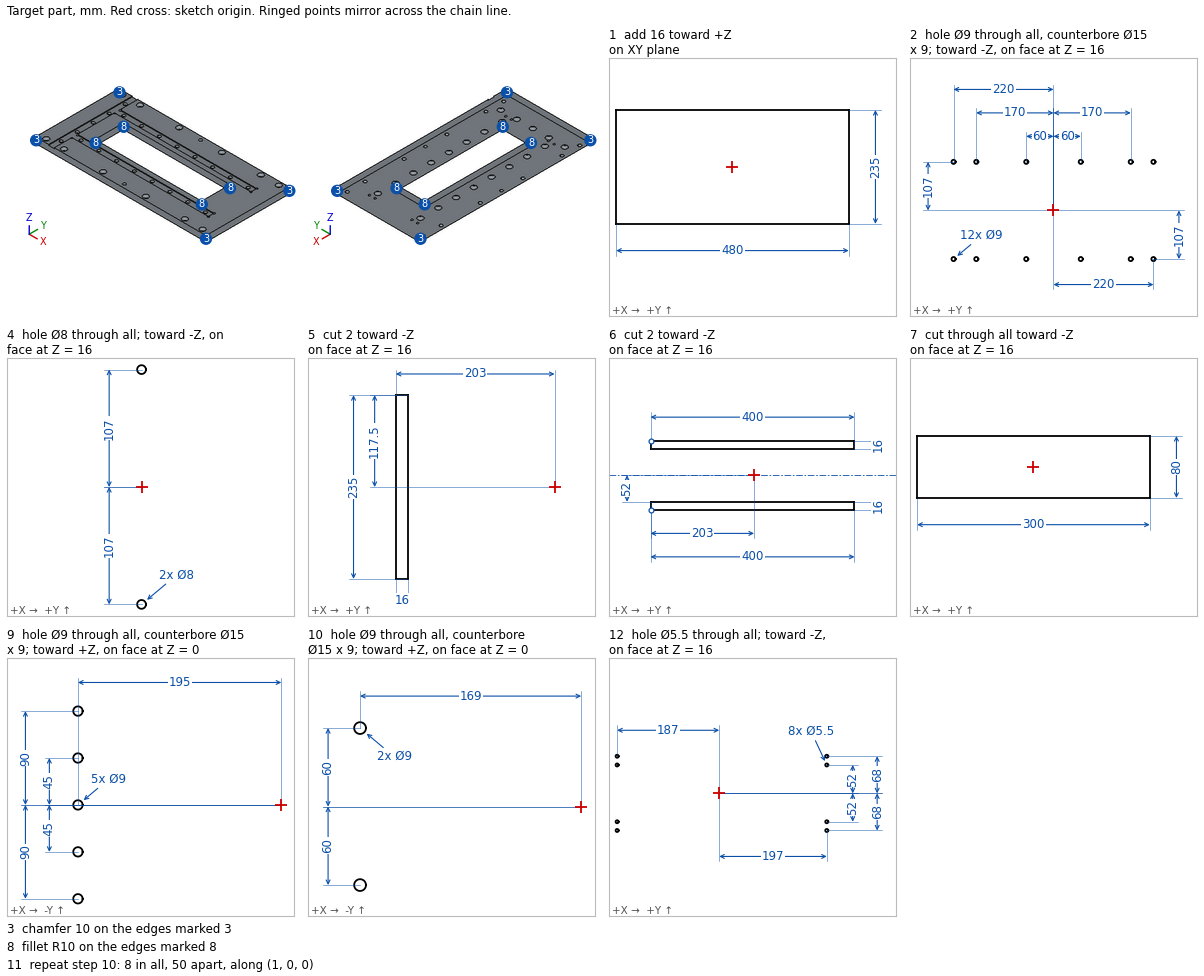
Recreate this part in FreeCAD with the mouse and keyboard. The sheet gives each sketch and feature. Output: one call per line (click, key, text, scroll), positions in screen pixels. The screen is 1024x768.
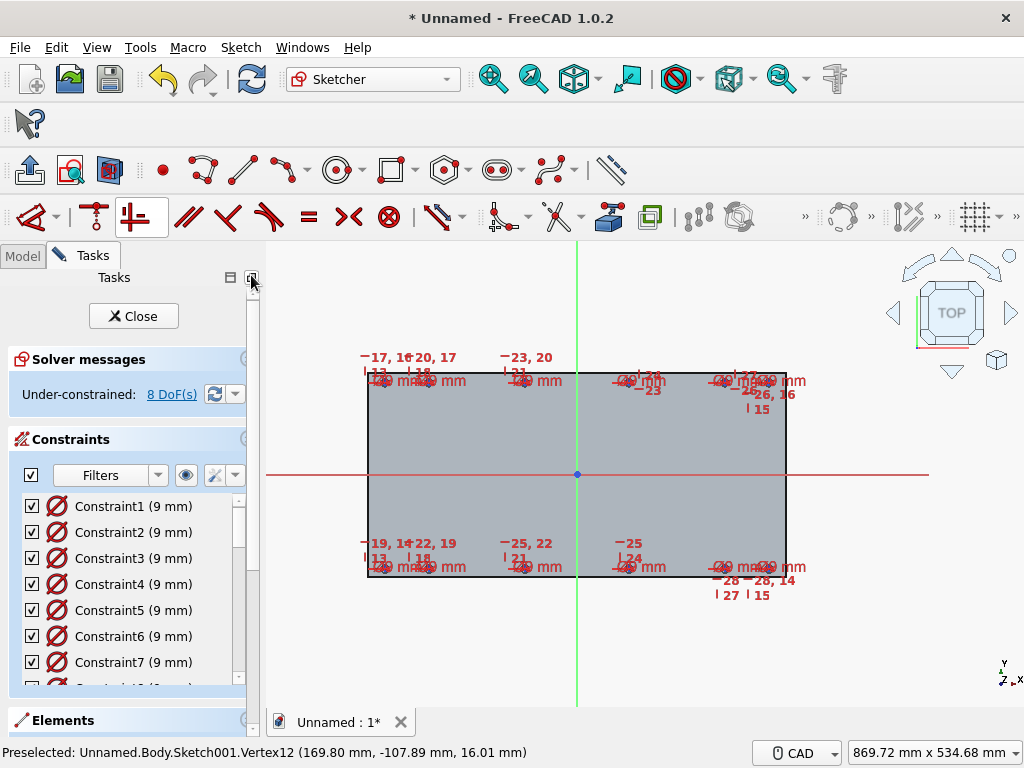
click(32, 218)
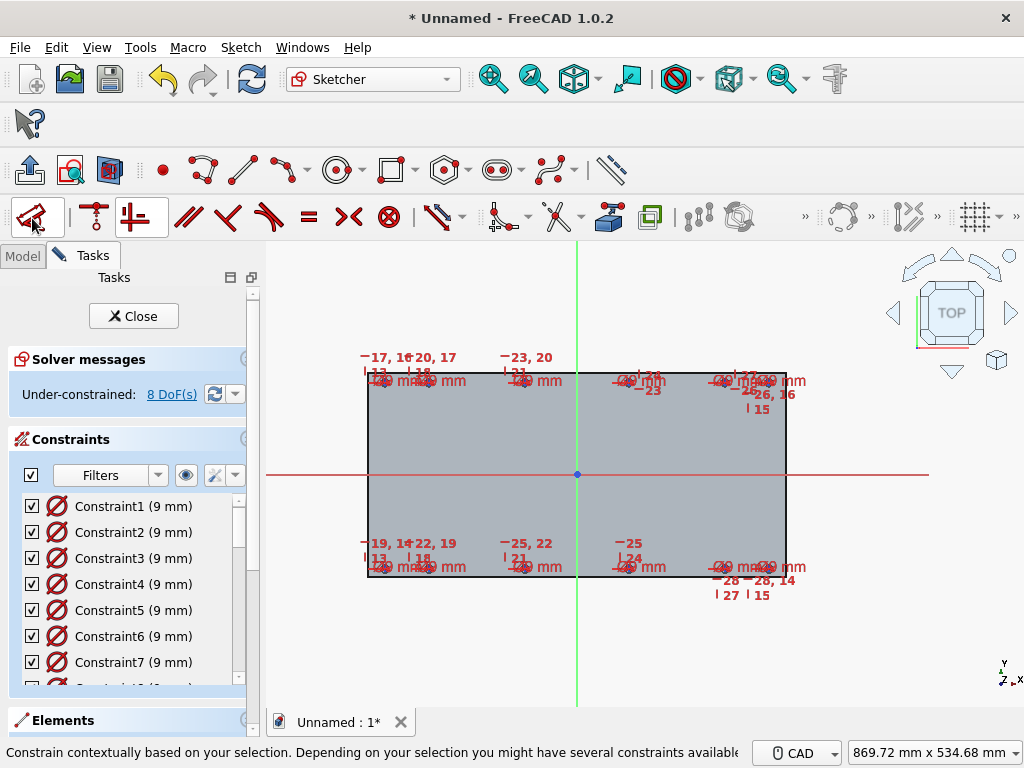
click(525, 383)
click(551, 349)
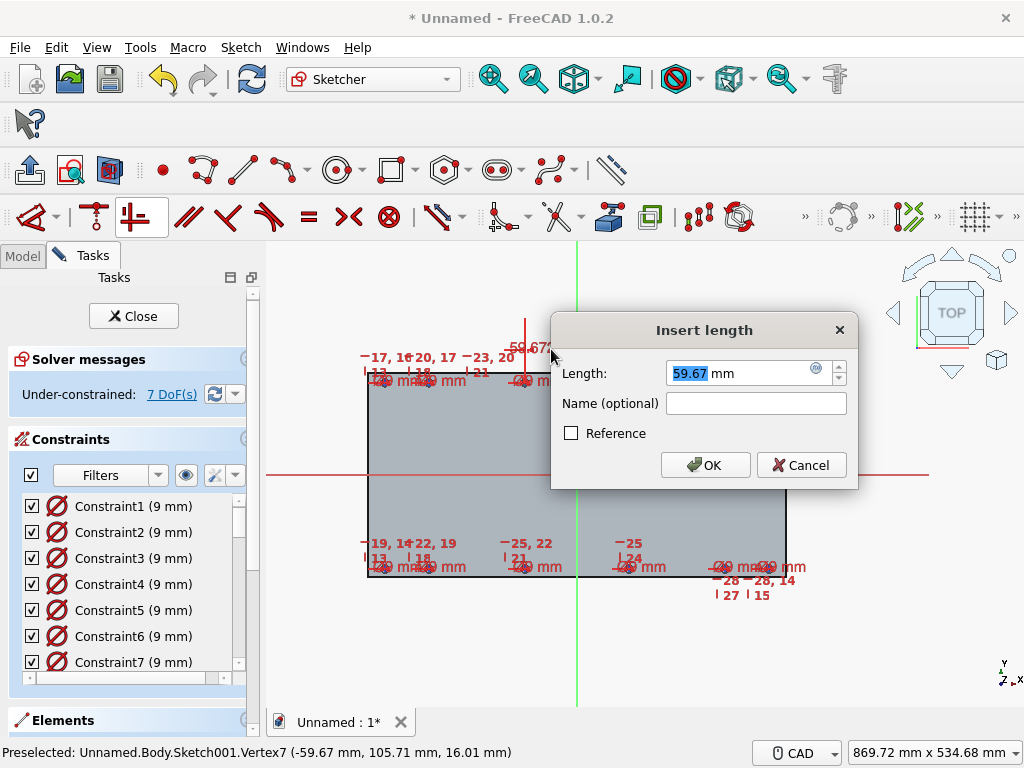
text(60)
key(Return)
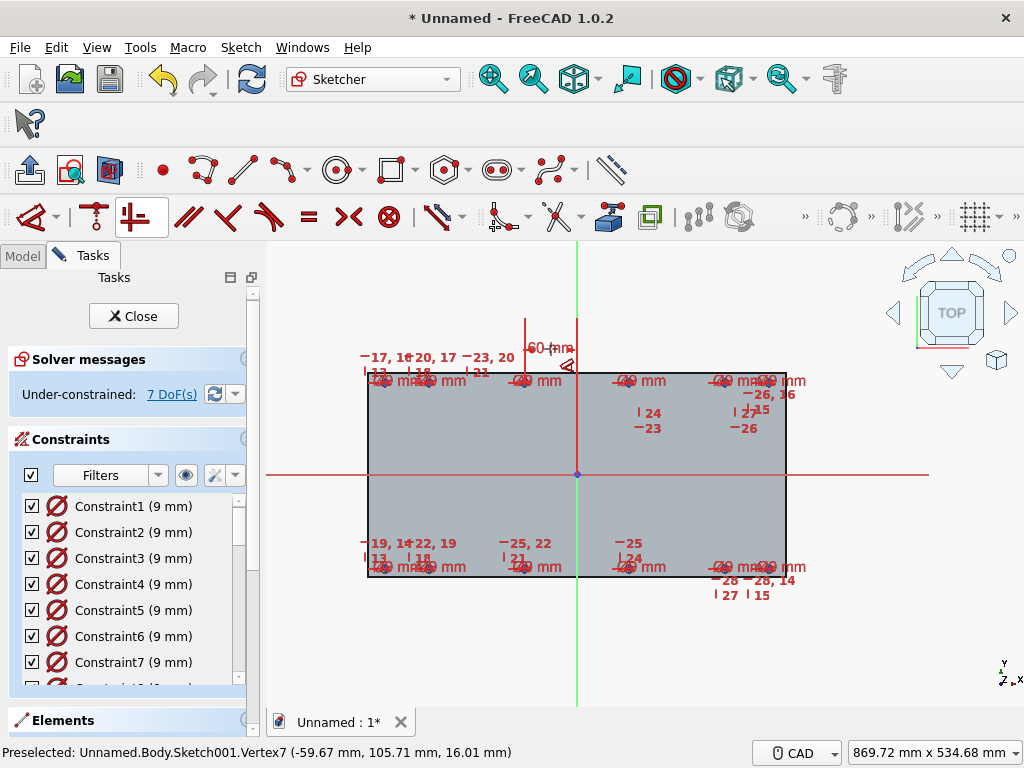
click(629, 383)
click(621, 349)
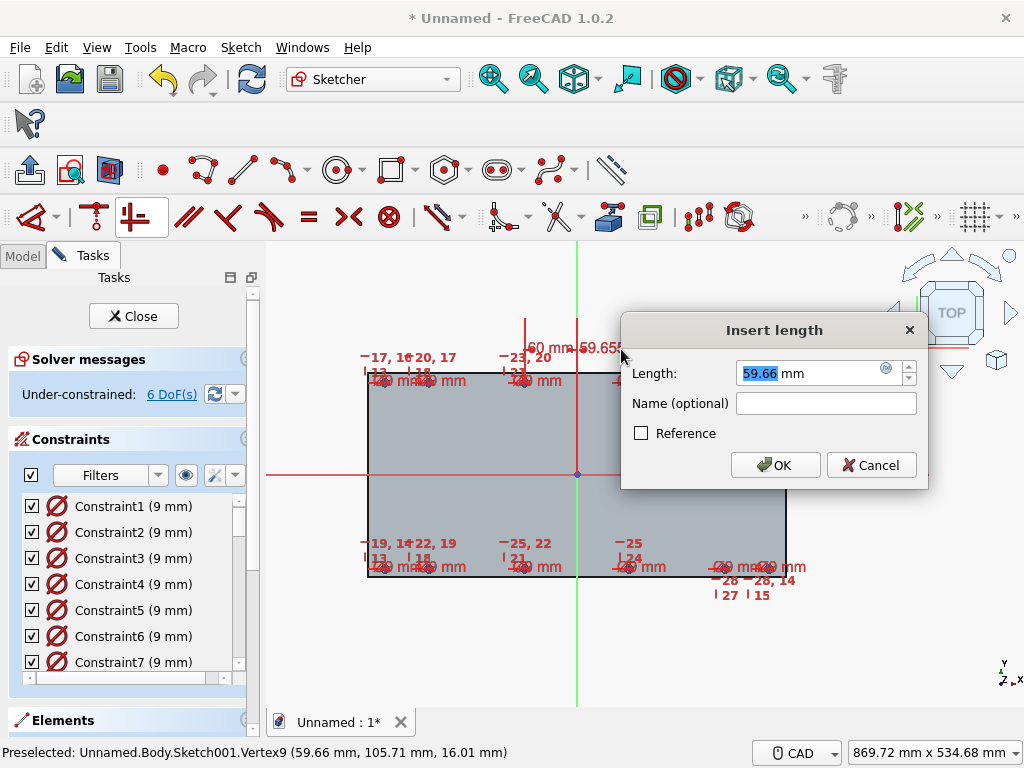
text(60)
key(Return)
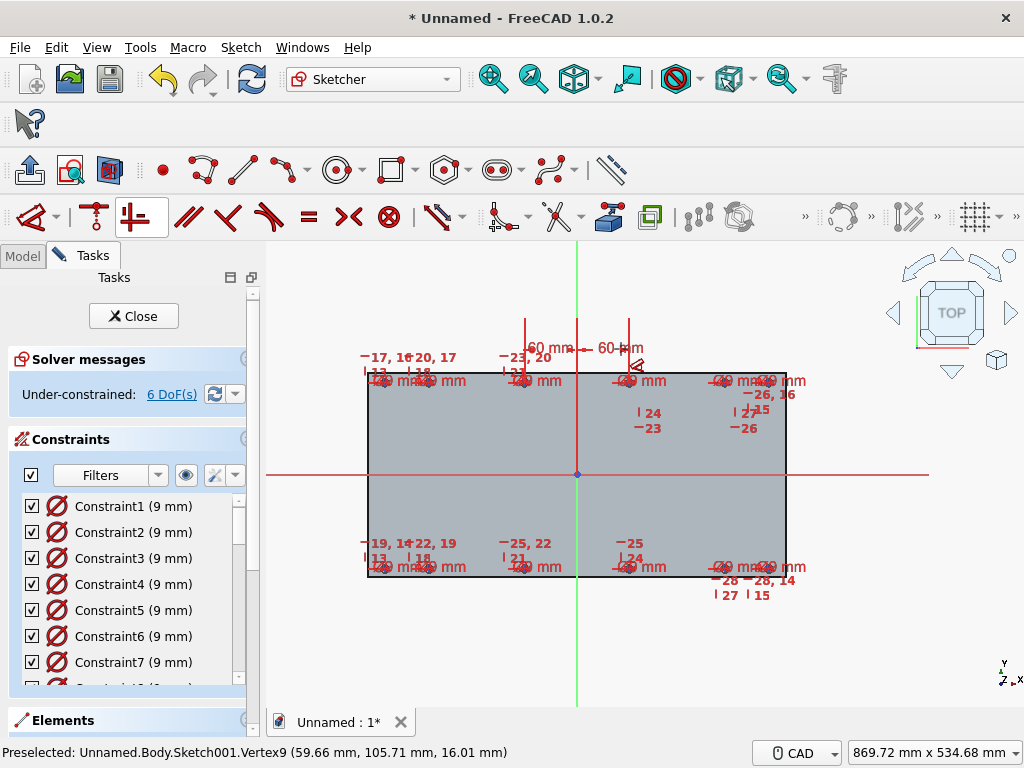
click(385, 383)
click(437, 349)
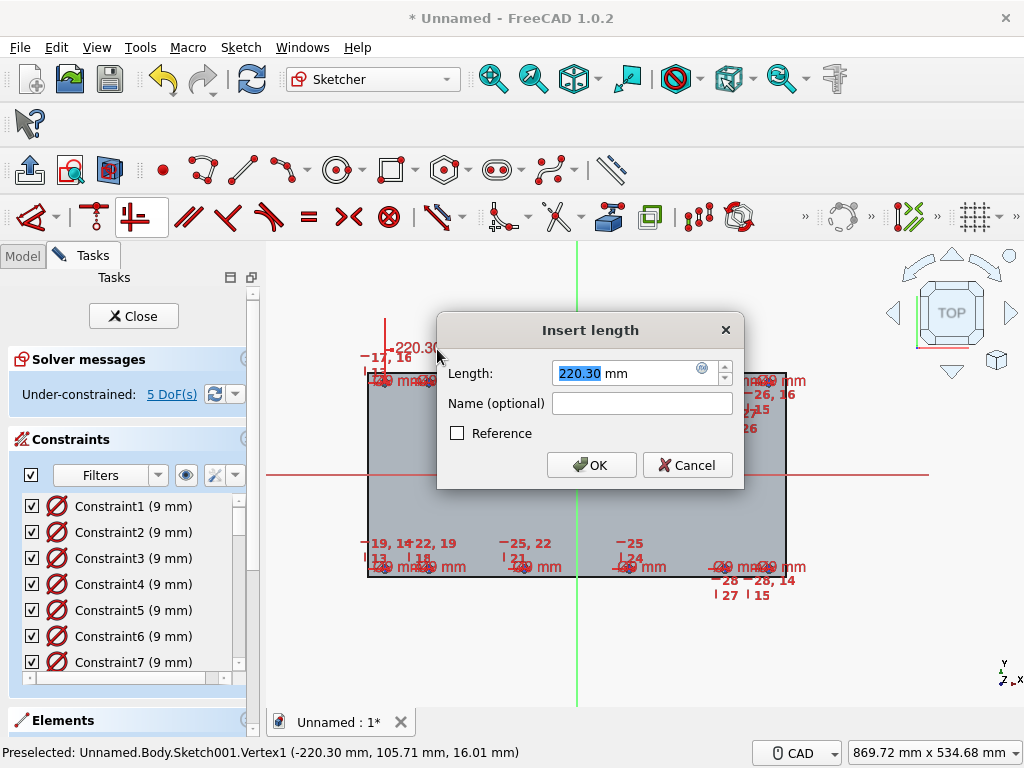
text(220)
key(Return)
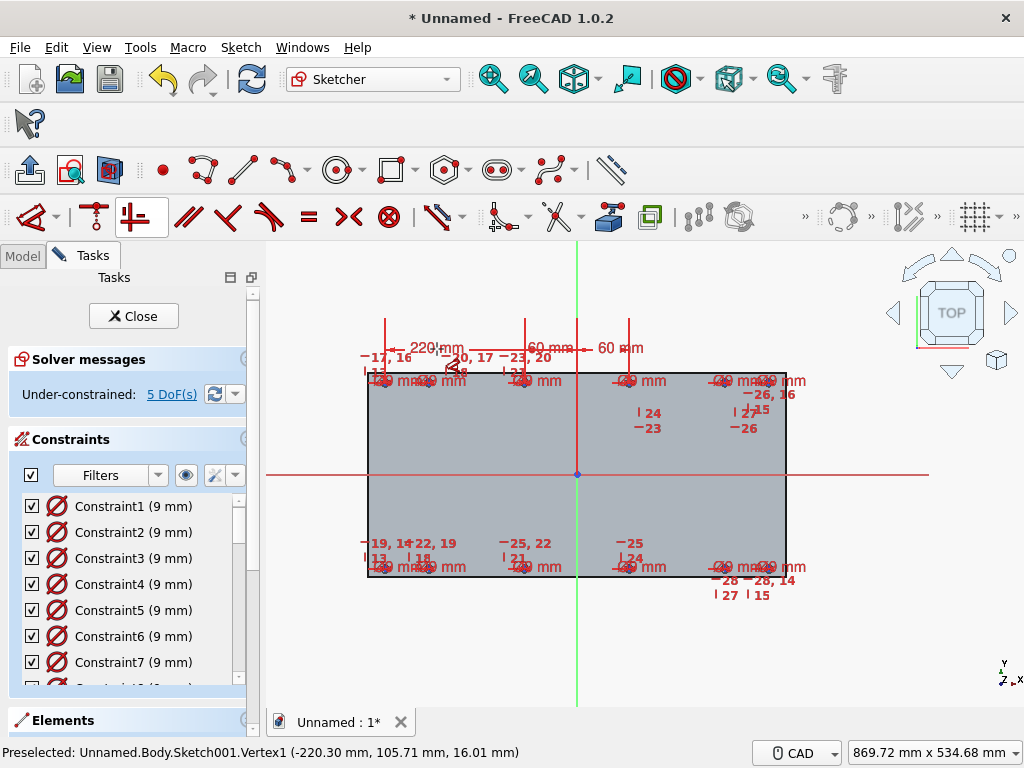
click(385, 383)
click(351, 429)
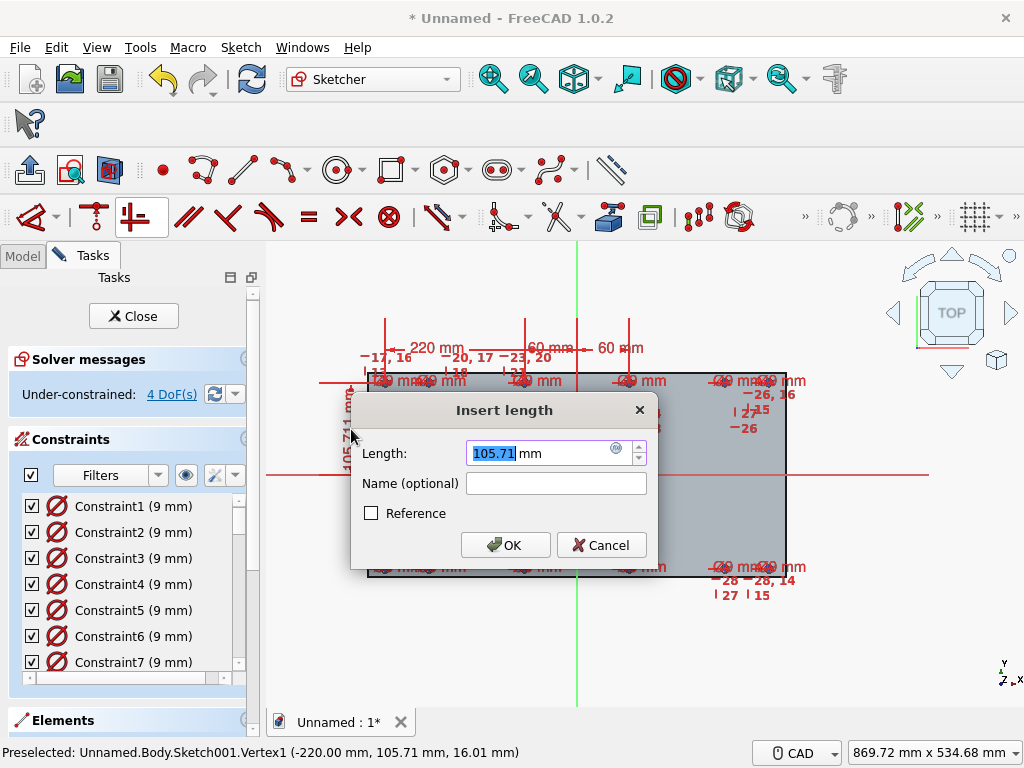
text(107)
key(Return)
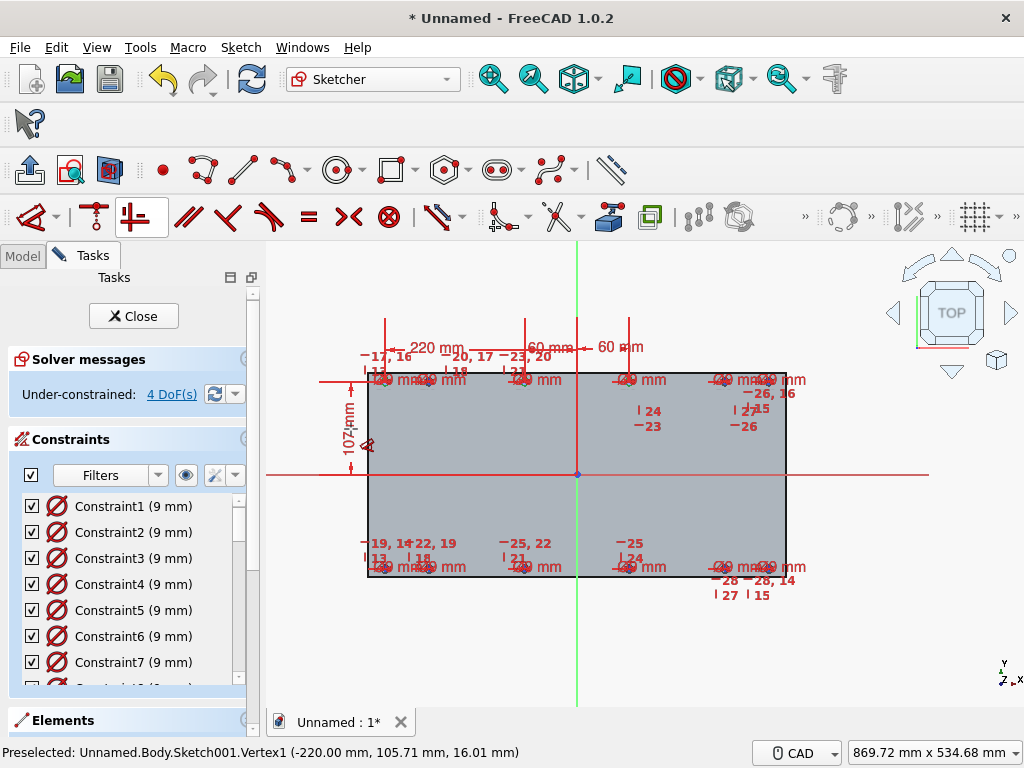
click(769, 569)
click(673, 603)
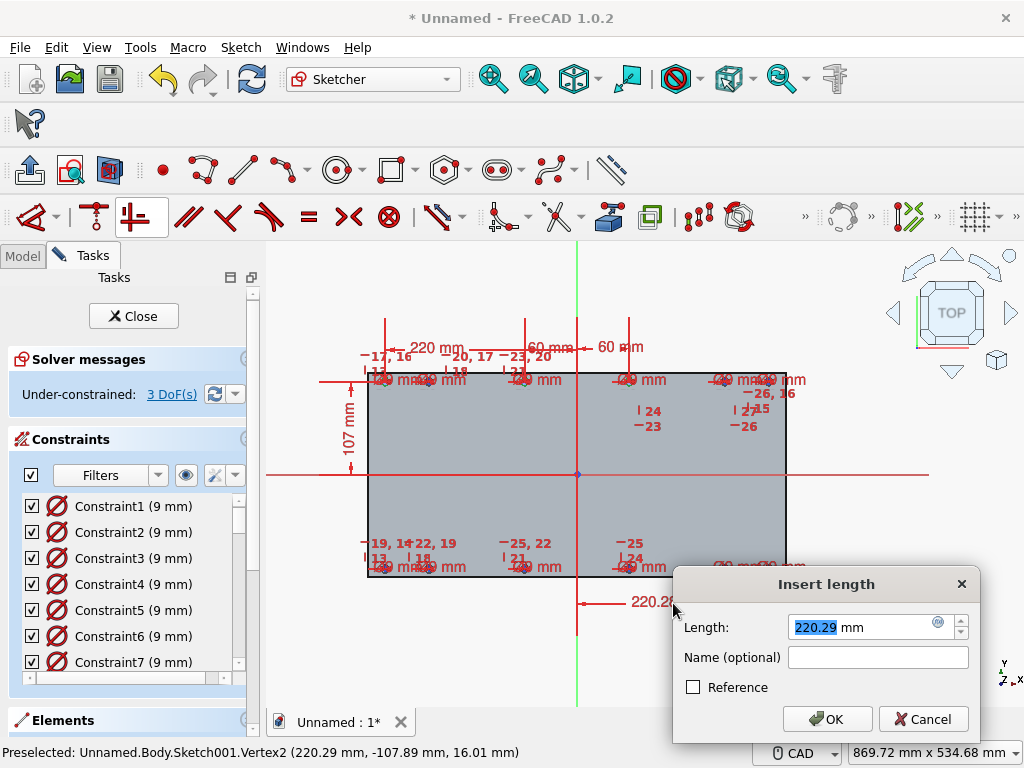
text(220)
key(Return)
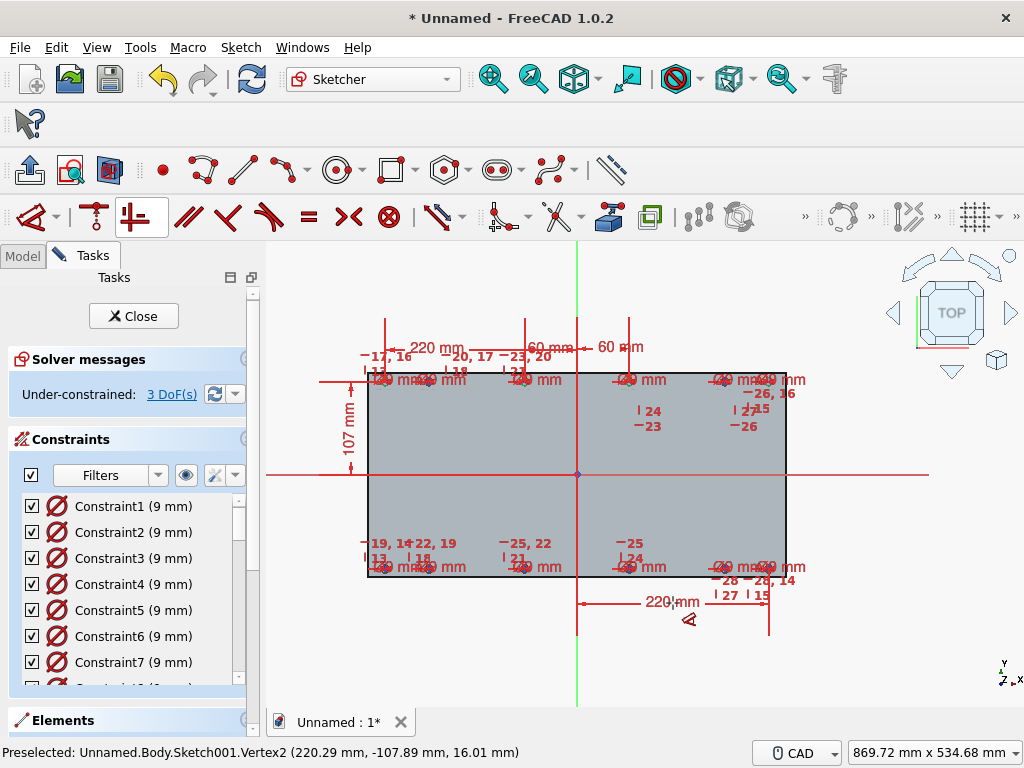
click(769, 569)
click(803, 522)